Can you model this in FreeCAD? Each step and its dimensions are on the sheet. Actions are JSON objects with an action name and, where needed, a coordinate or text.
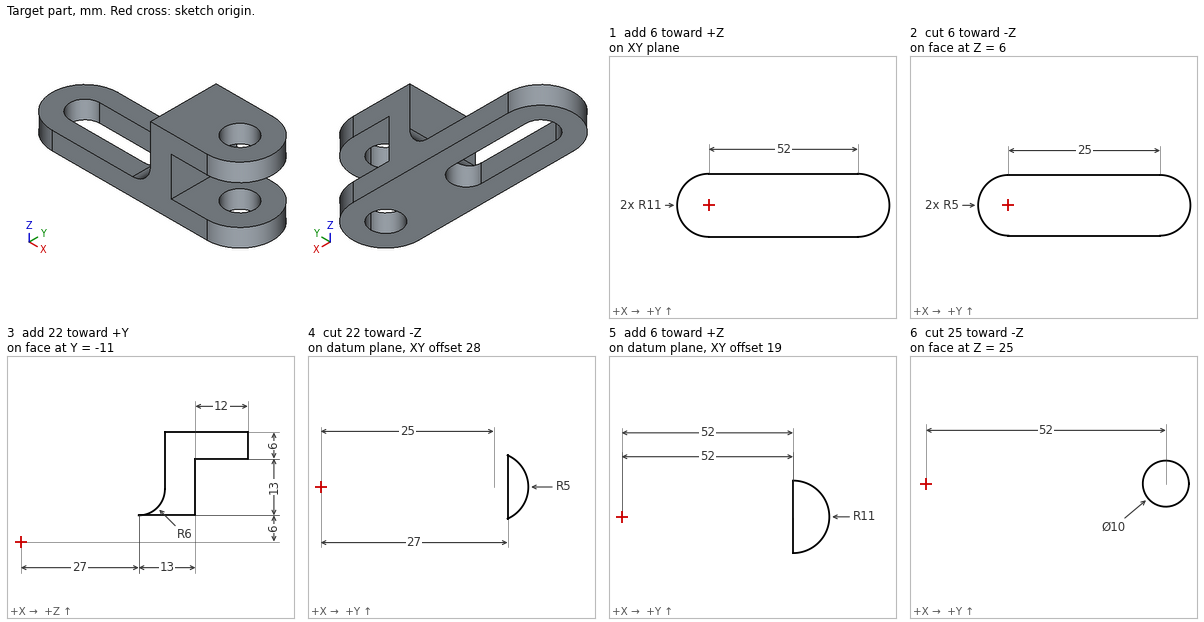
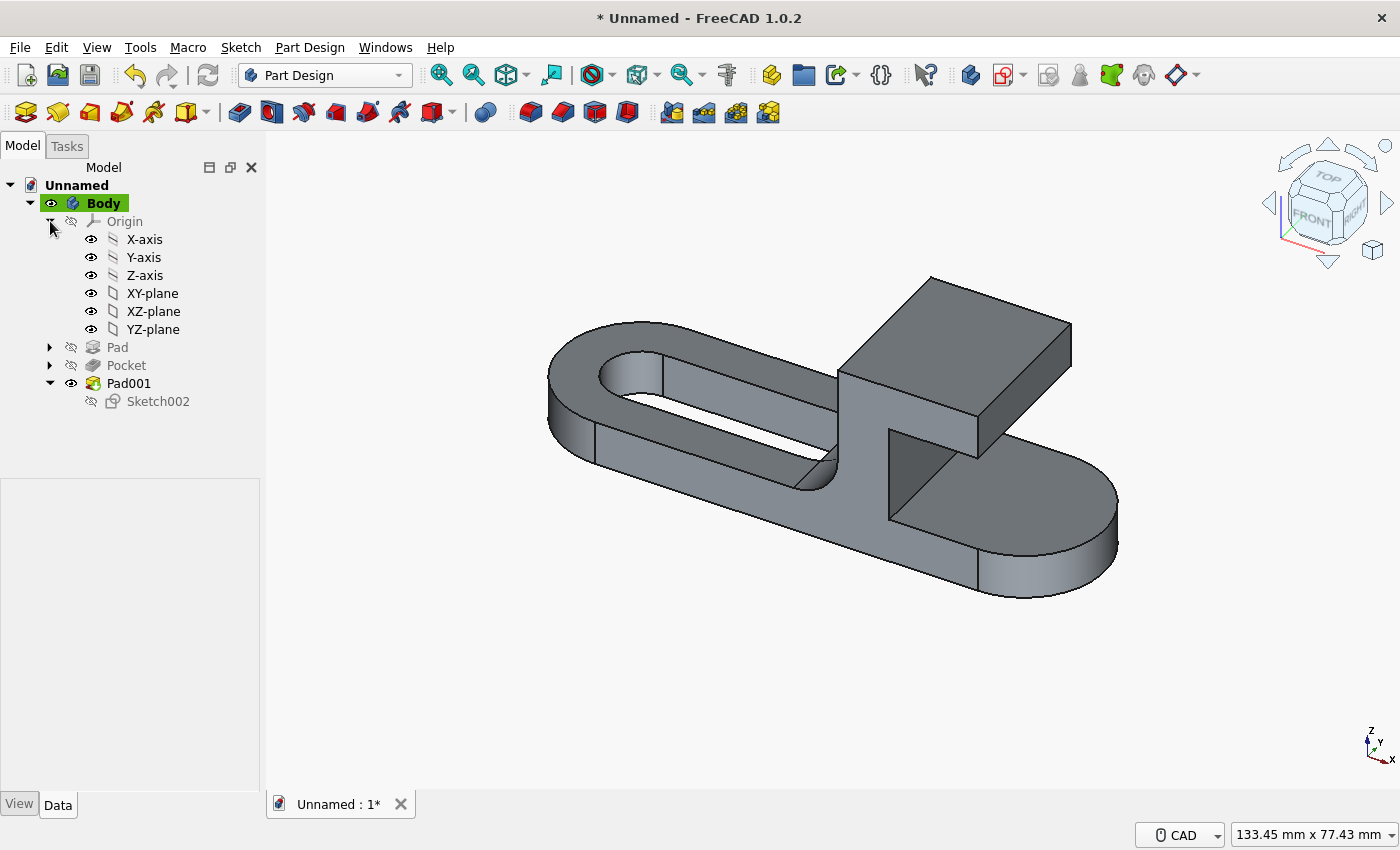
{"action": "left_click", "coordinate": [136, 293]}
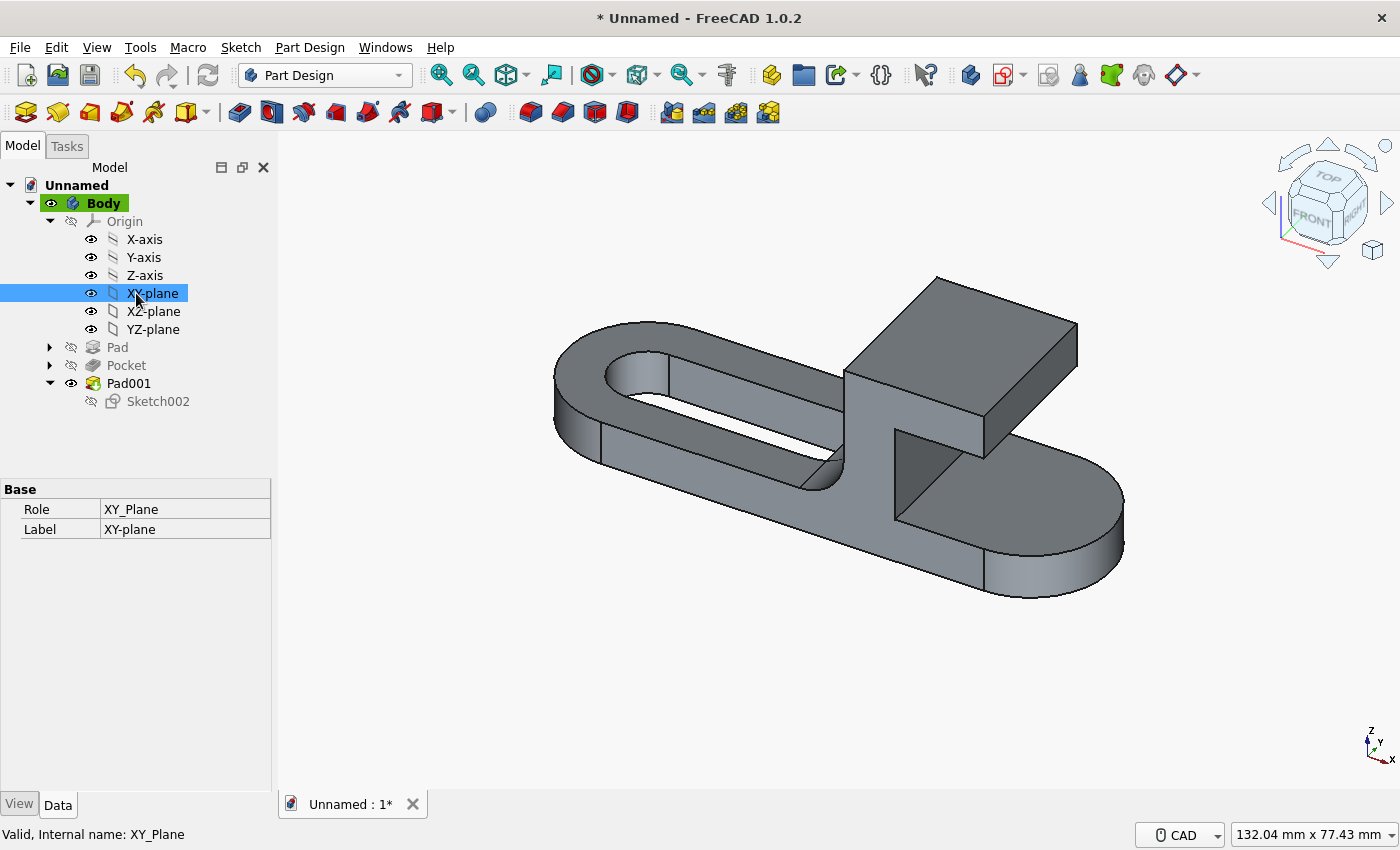
{"action": "left_click", "coordinate": [1176, 76]}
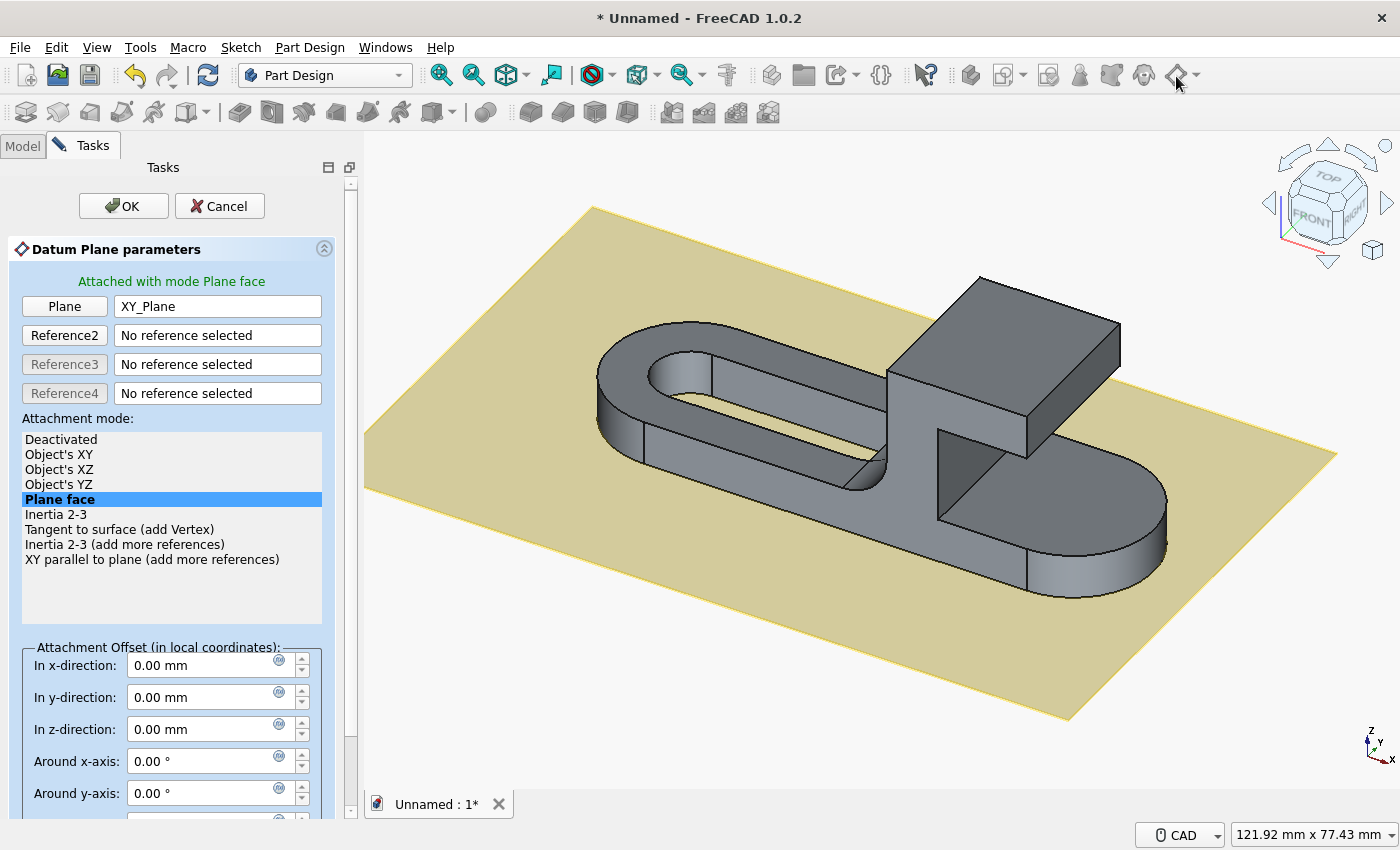
{"action": "triple_click", "coordinate": [210, 729]}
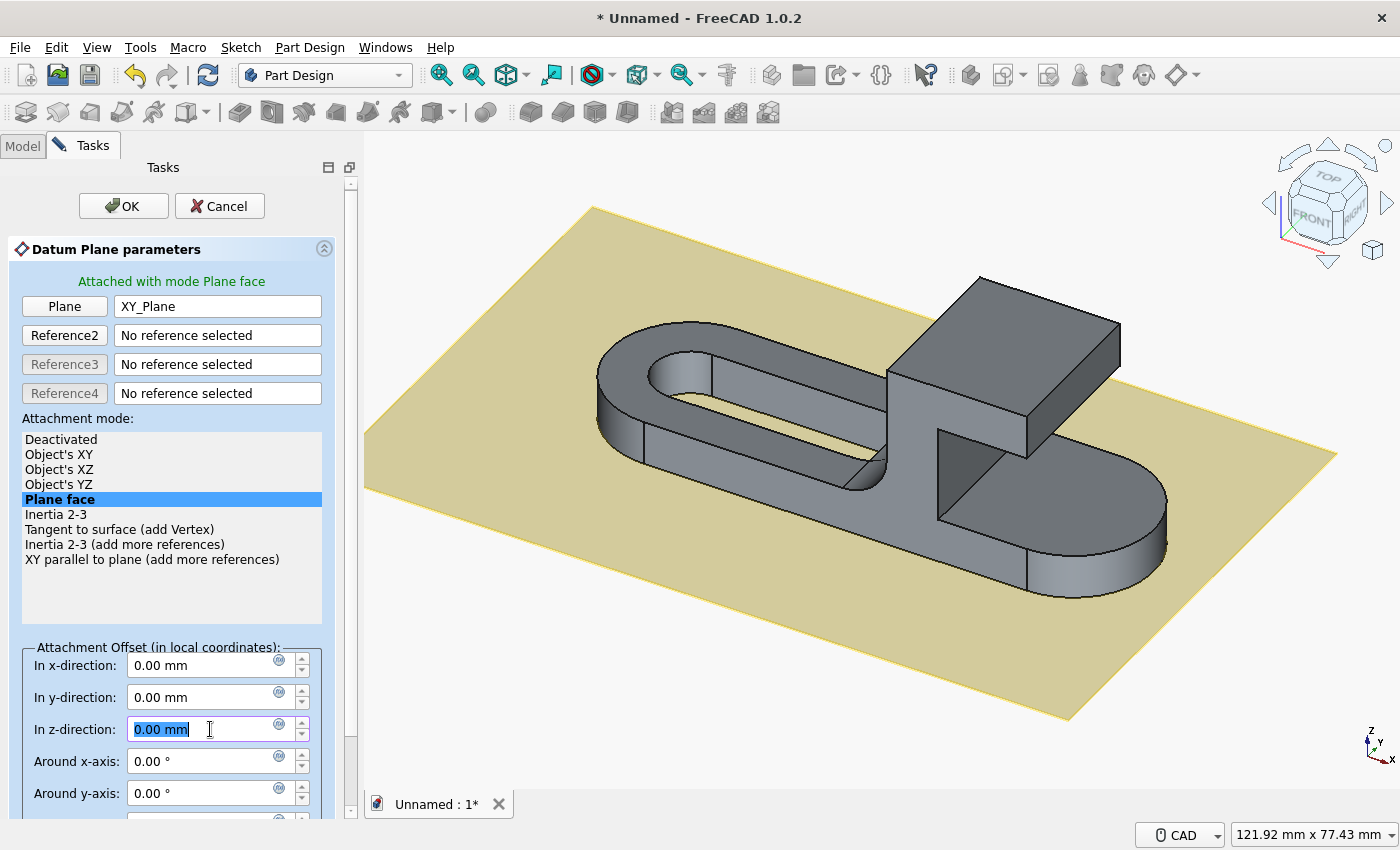
{"action": "type", "text": "28"}
{"action": "key", "text": "Tab"}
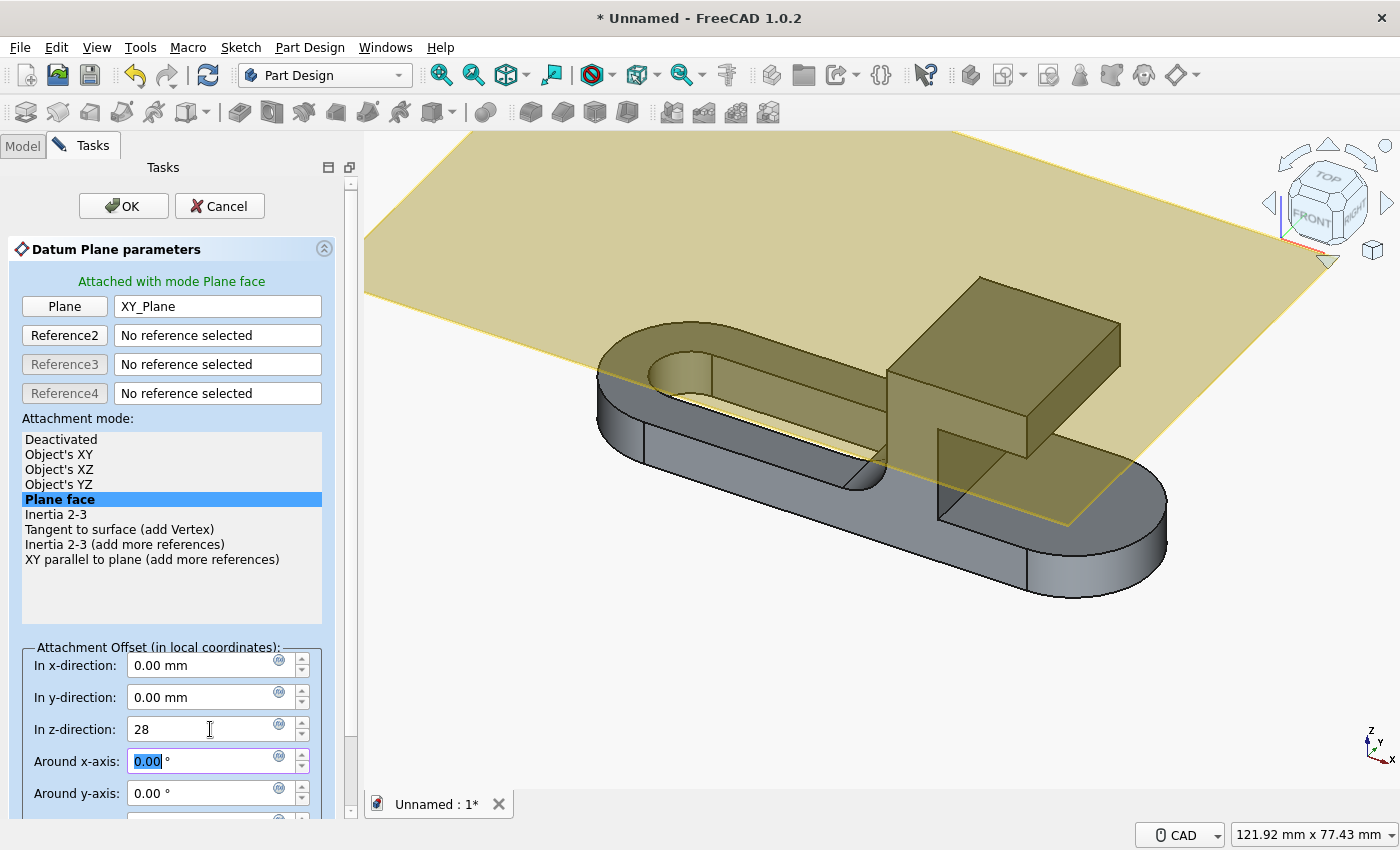
{"action": "left_click", "coordinate": [124, 206]}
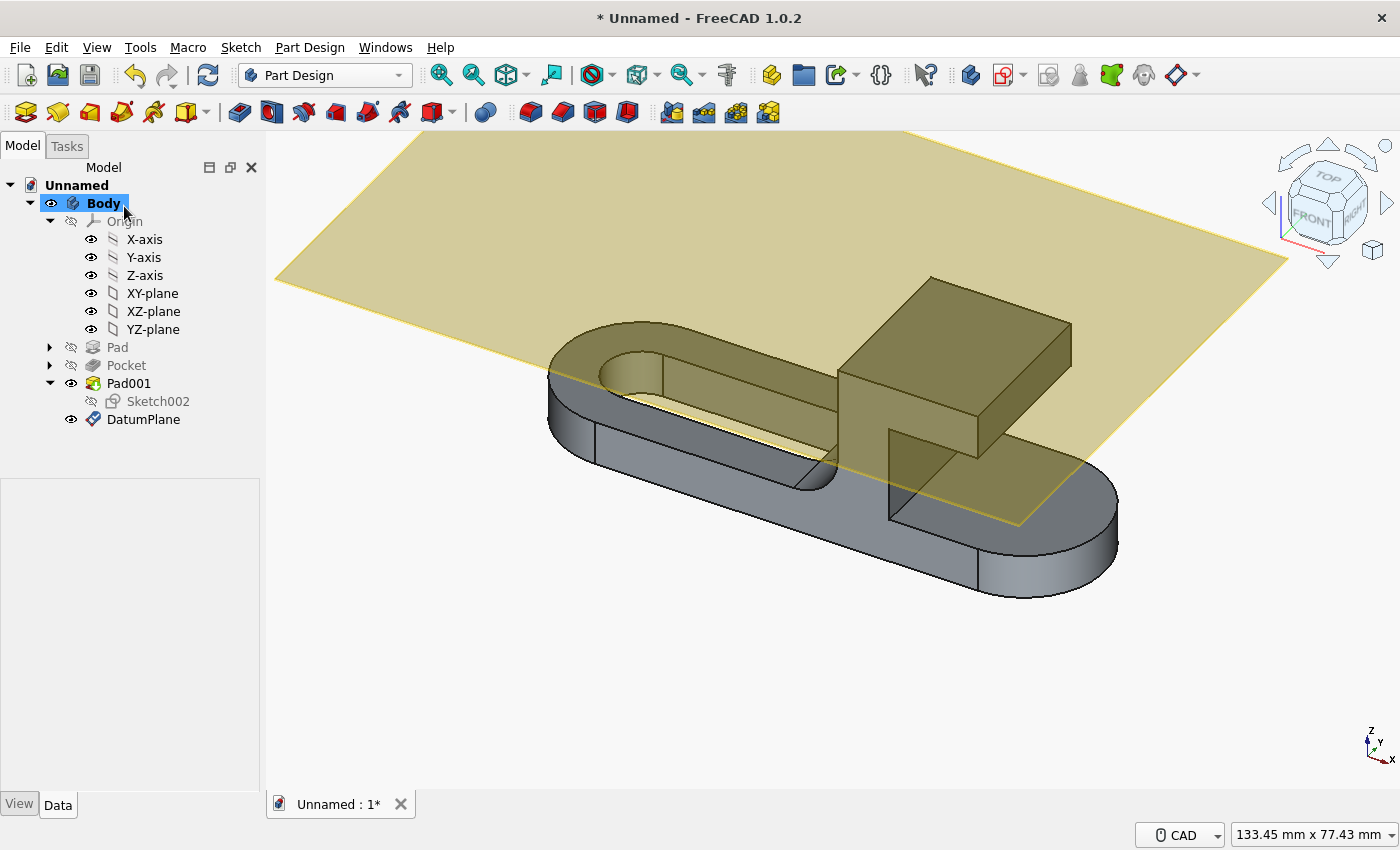
{"action": "left_click", "coordinate": [116, 419]}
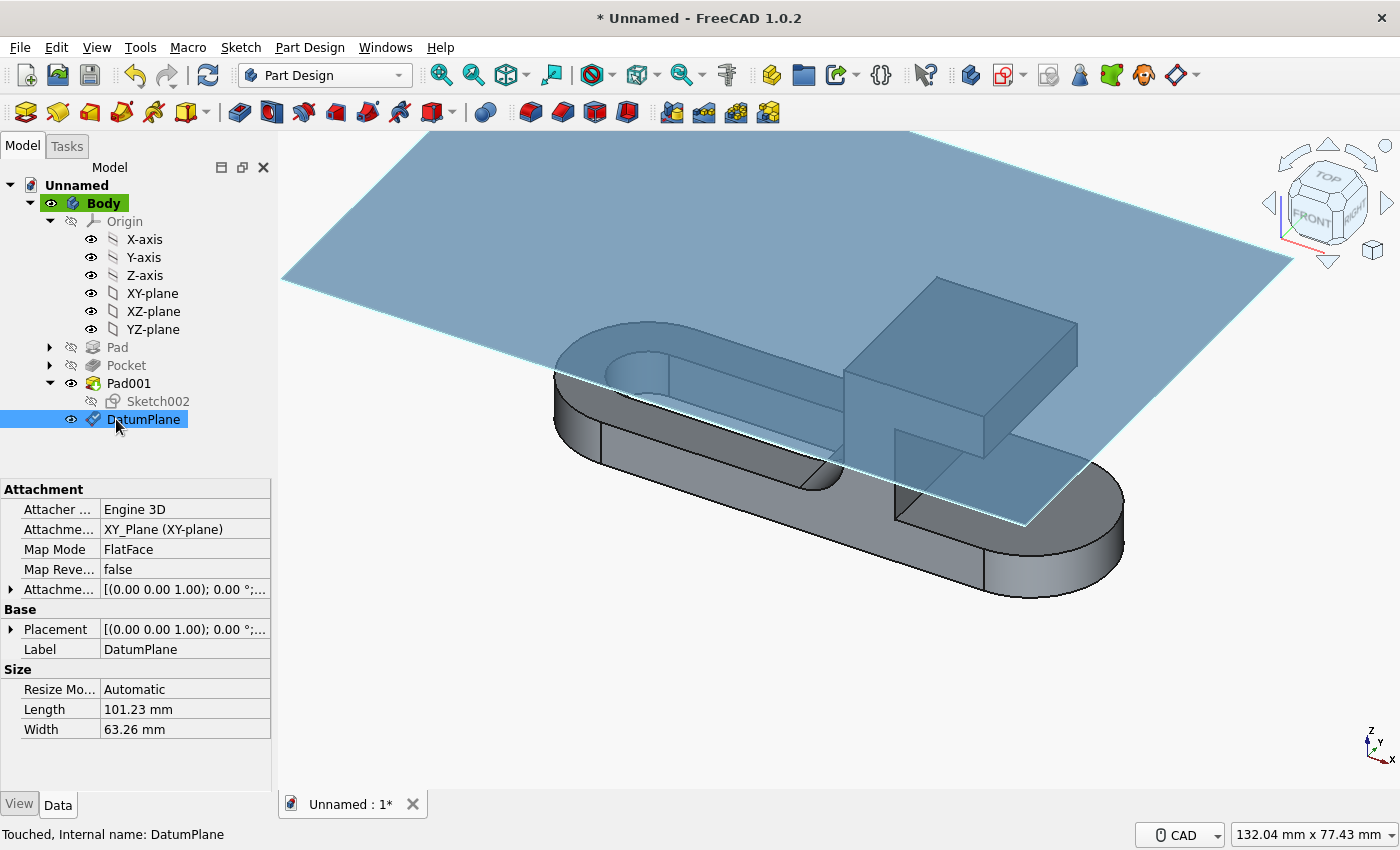
{"action": "left_click", "coordinate": [1004, 76]}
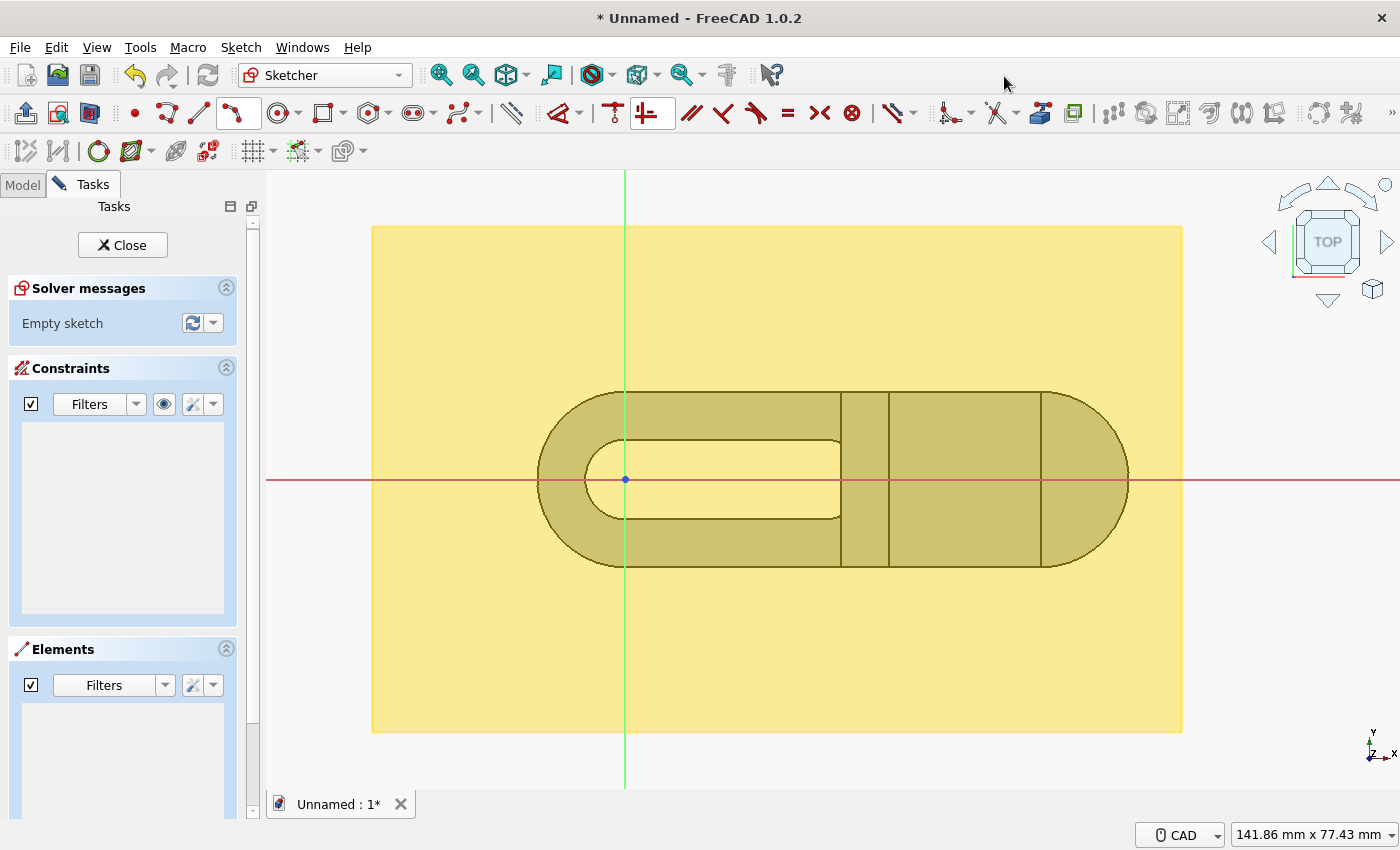
{"action": "scroll", "coordinate": [875, 479], "scroll_direction": "up", "scroll_amount": 8}